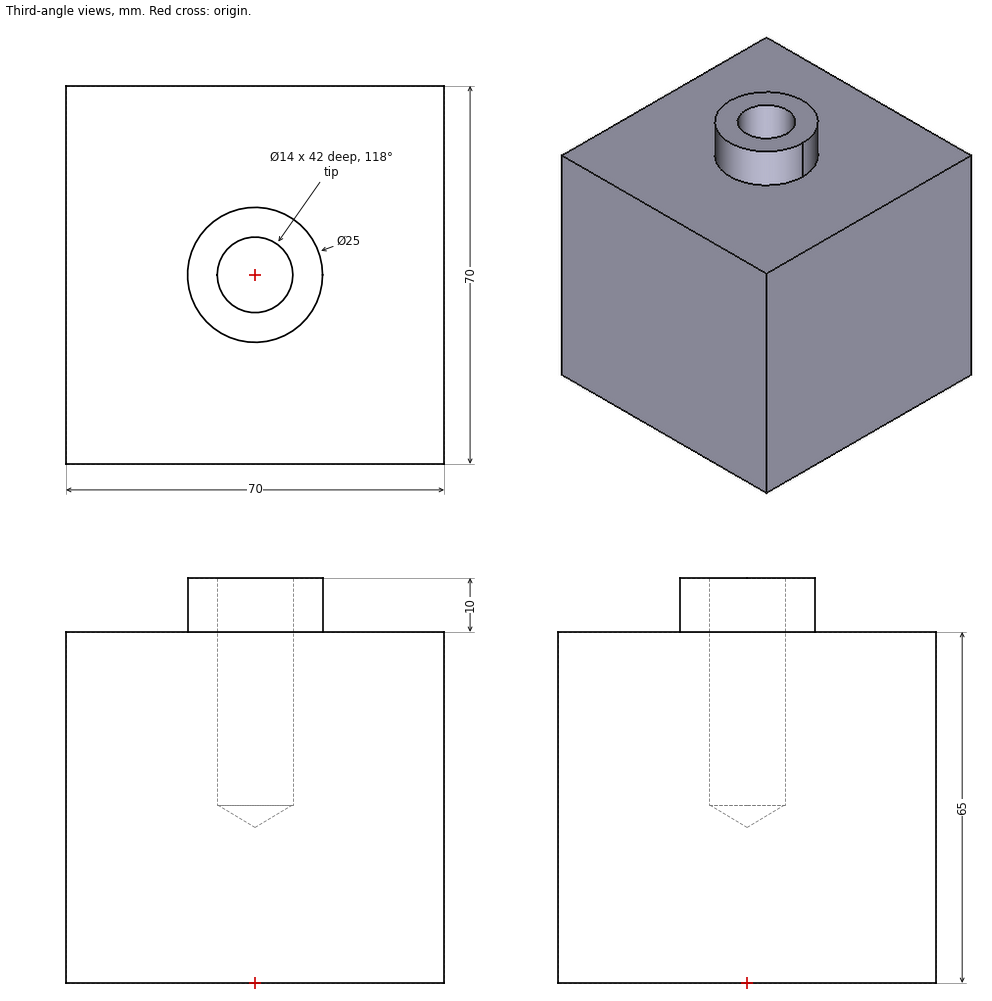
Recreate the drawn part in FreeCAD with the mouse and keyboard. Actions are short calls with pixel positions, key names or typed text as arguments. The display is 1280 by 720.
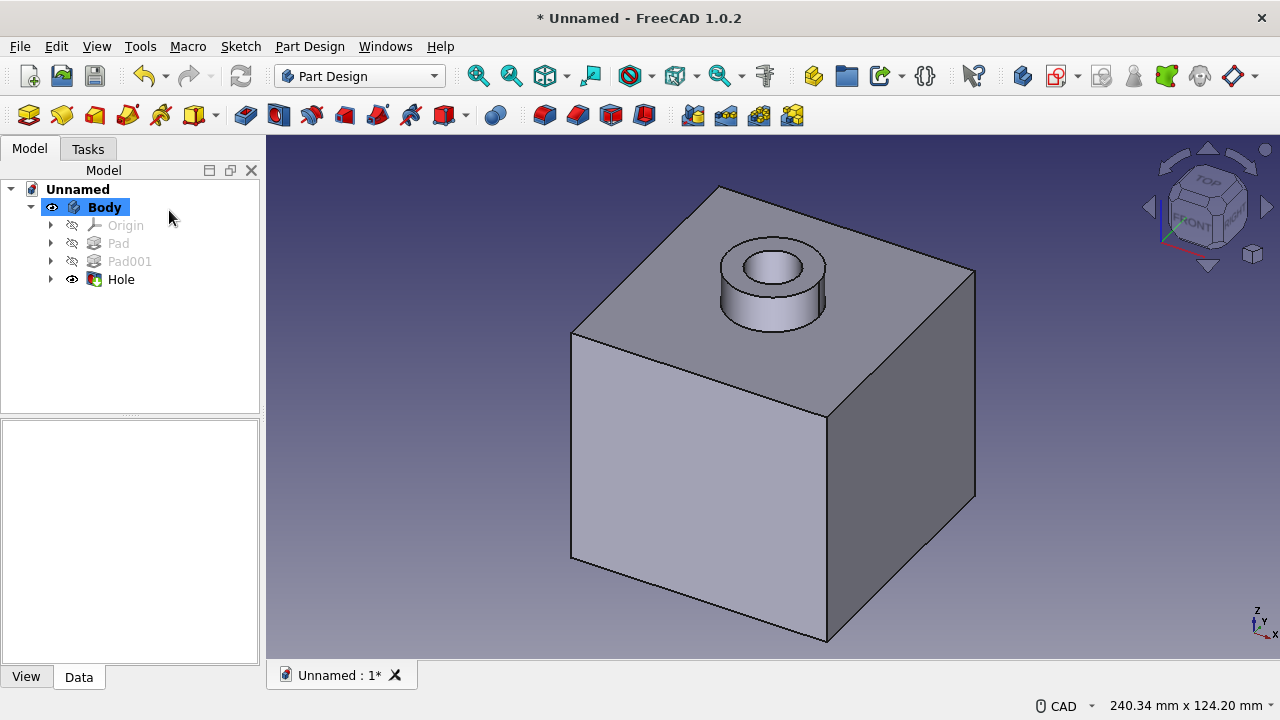
key(0)